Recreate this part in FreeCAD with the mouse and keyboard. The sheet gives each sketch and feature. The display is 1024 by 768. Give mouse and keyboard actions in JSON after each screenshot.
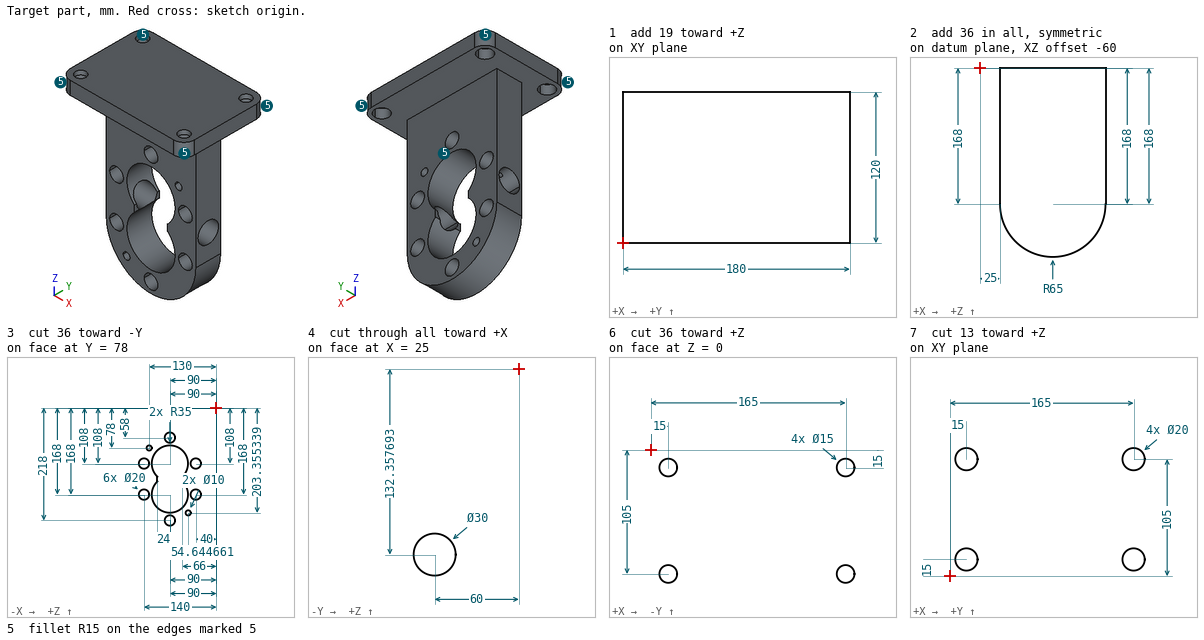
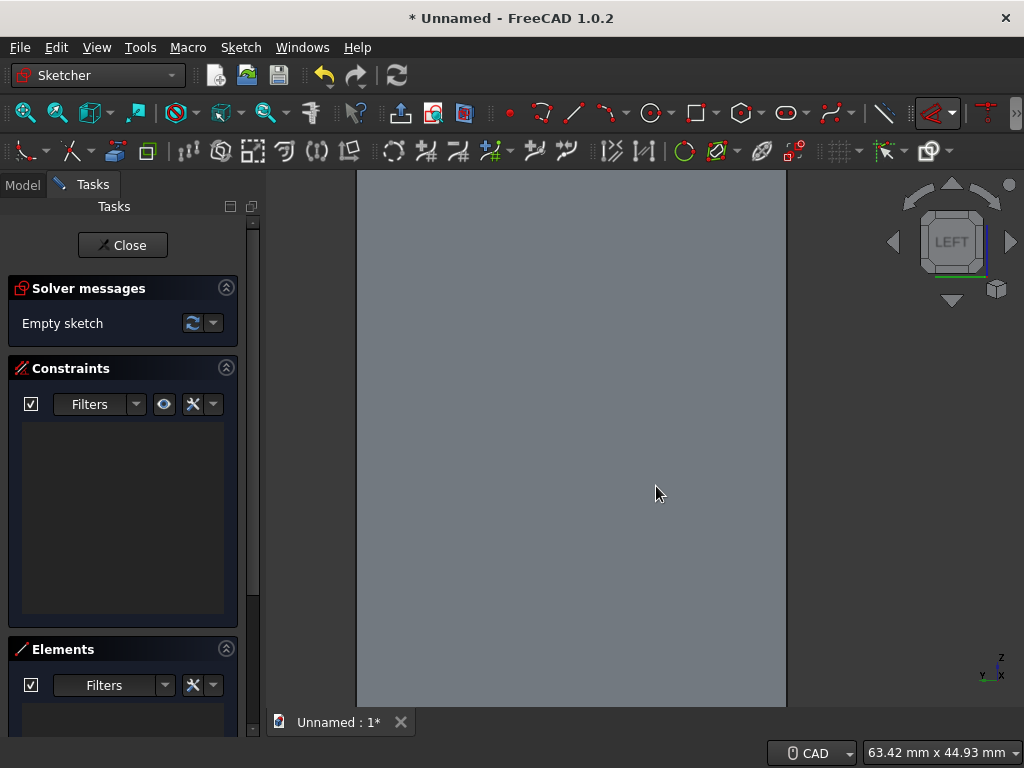
{"action": "left_click", "coordinate": [652, 114]}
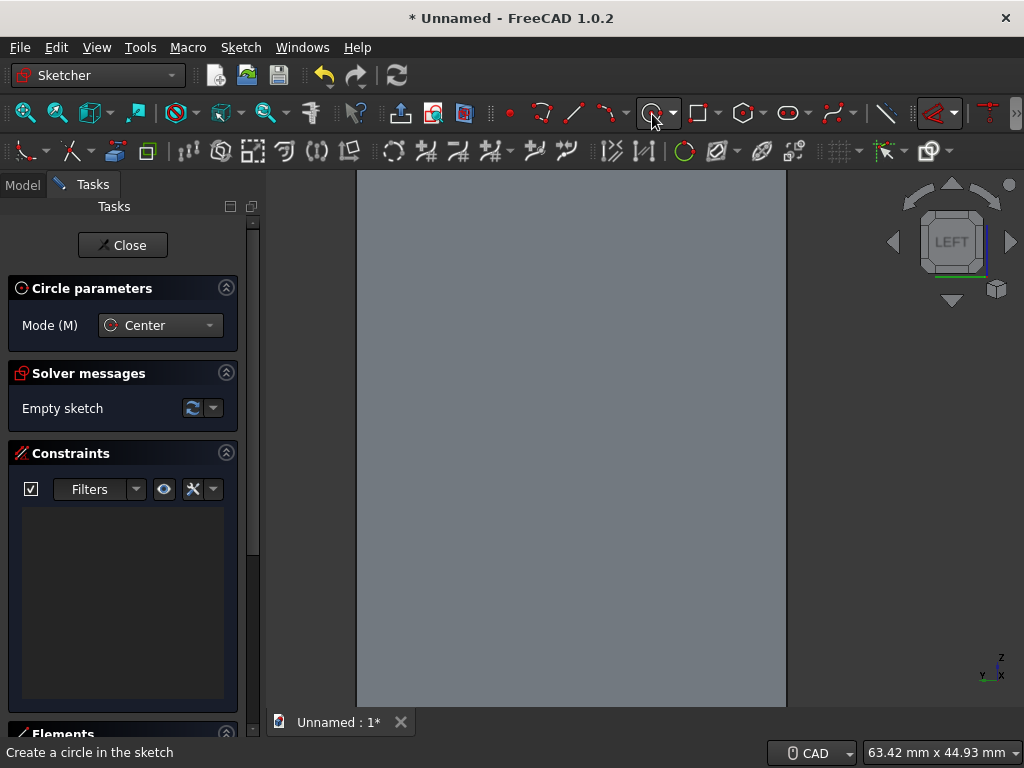
{"action": "left_click", "coordinate": [571, 435]}
{"action": "left_click", "coordinate": [698, 309]}
{"action": "key", "text": "Escape"}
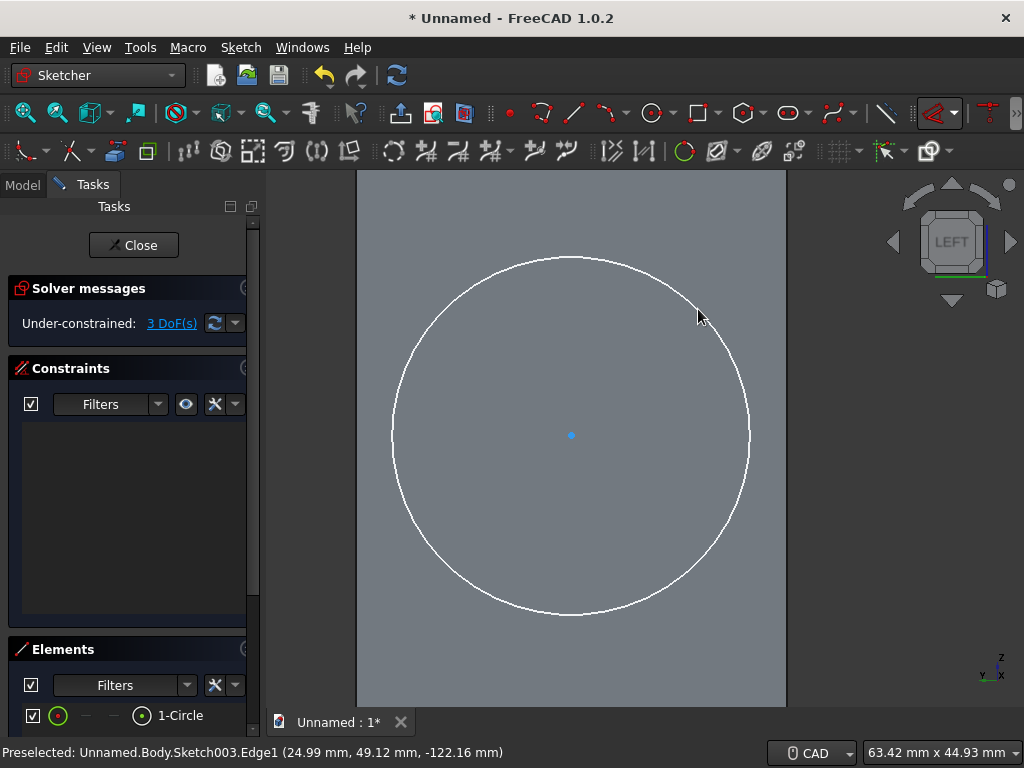
{"action": "left_click", "coordinate": [697, 309]}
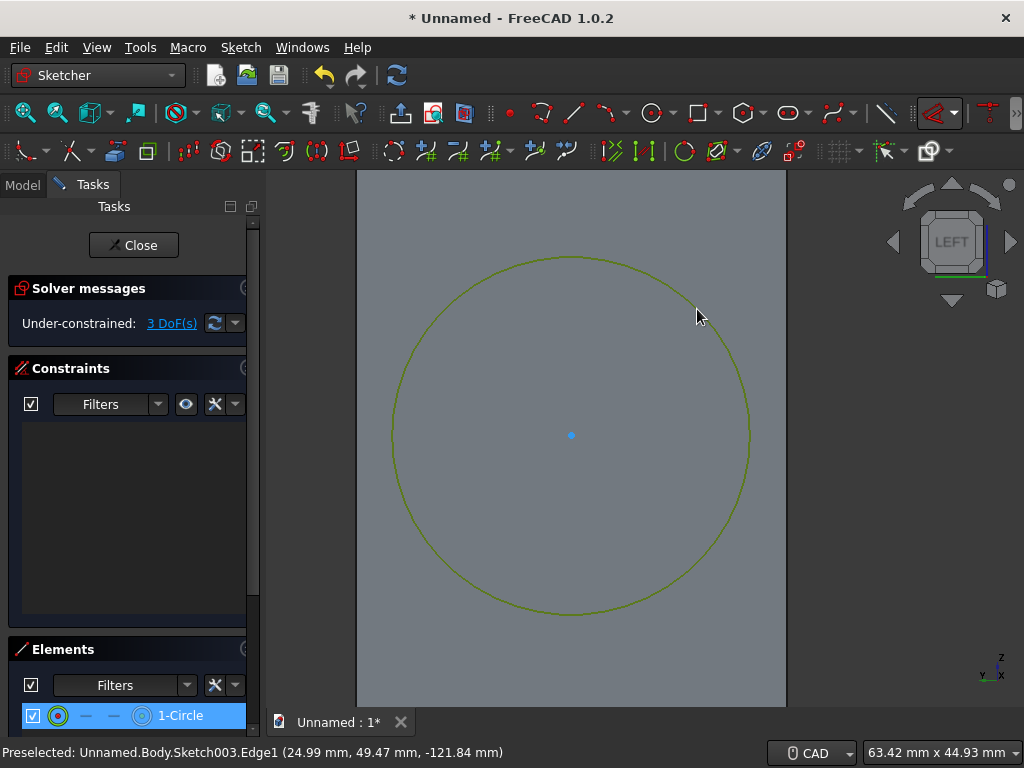
{"action": "left_click", "coordinate": [956, 114]}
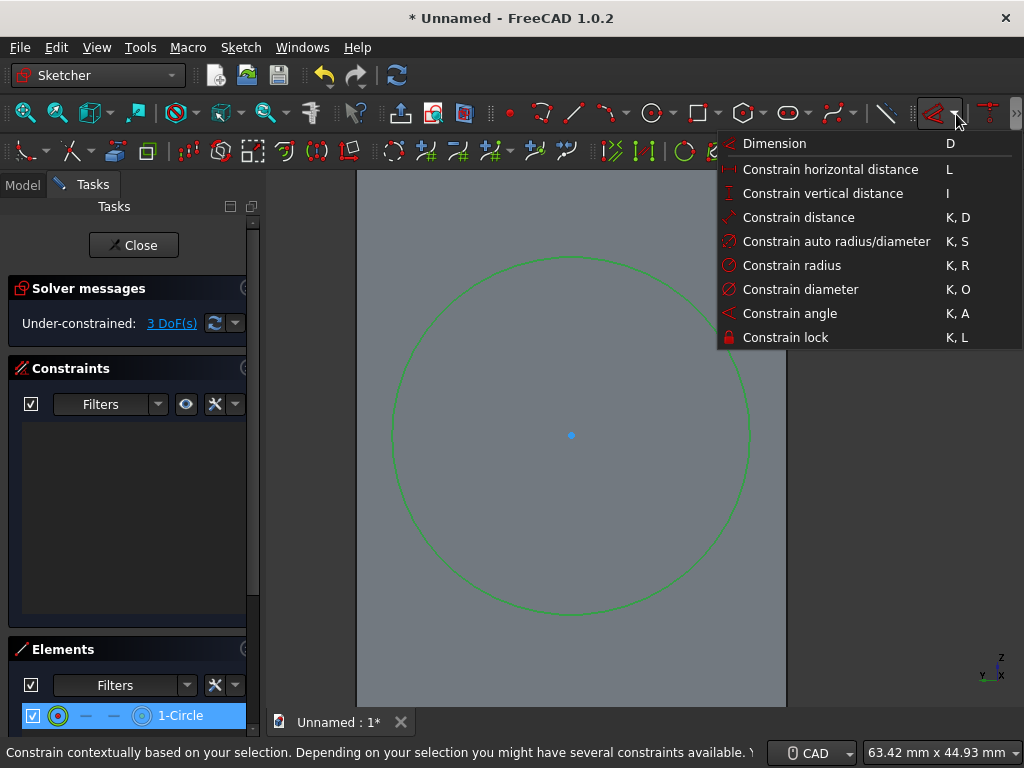
{"action": "left_click", "coordinate": [870, 289]}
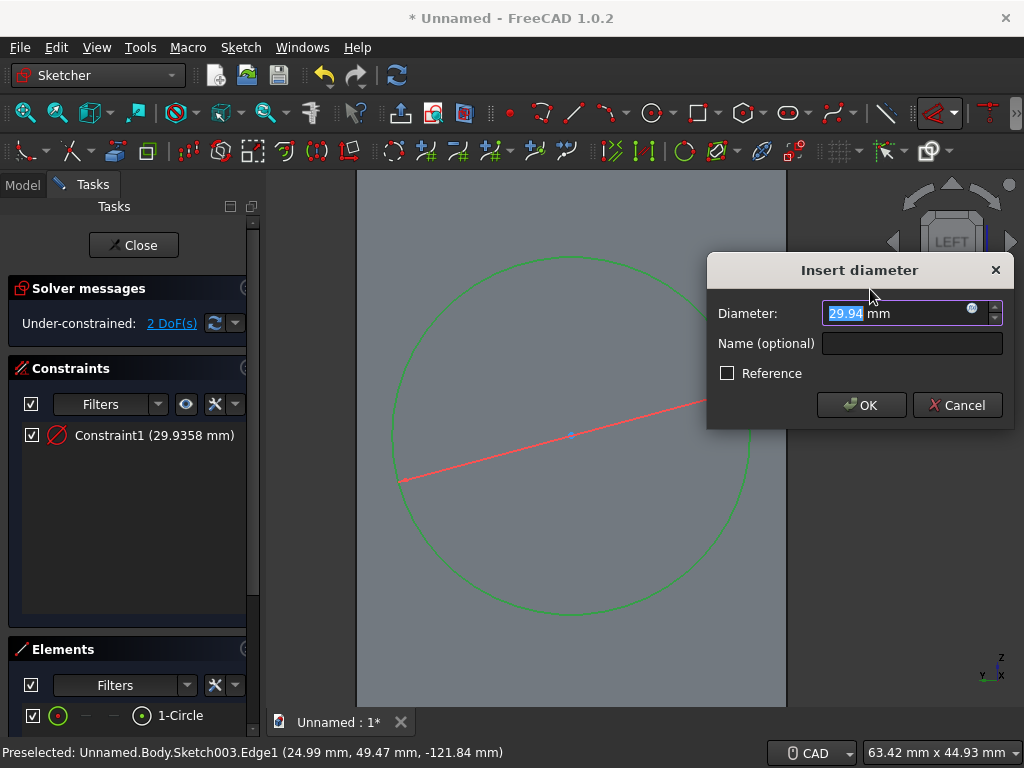
{"action": "type", "text": "30"}
{"action": "key", "text": "Return"}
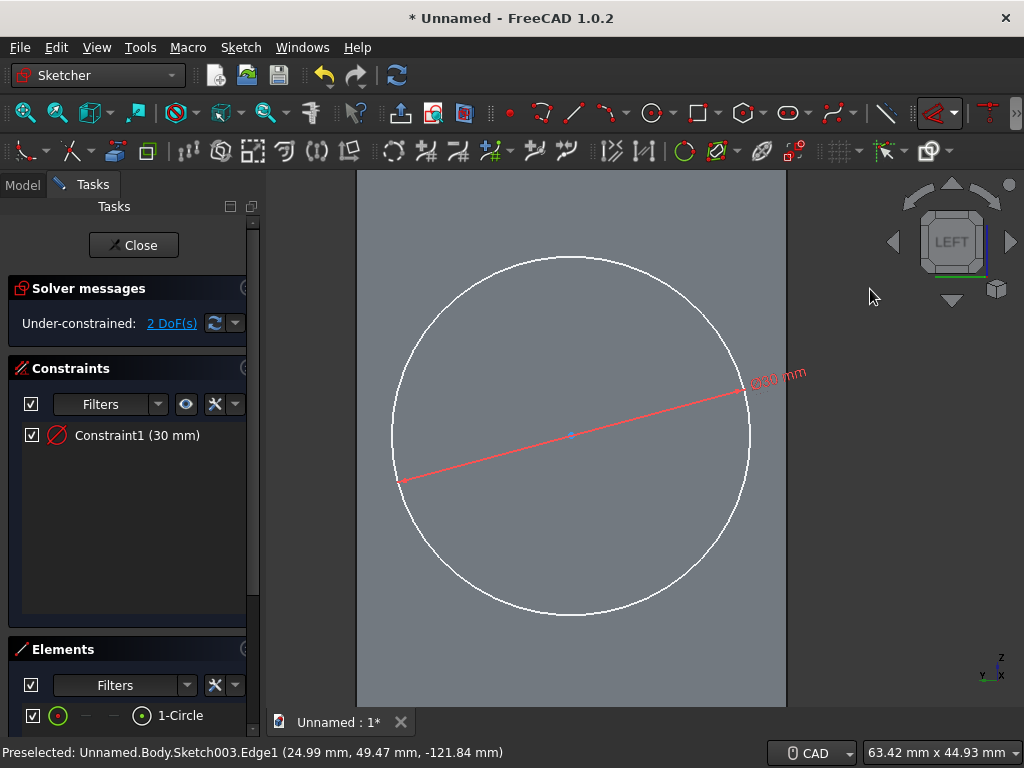
{"action": "left_click", "coordinate": [571, 436]}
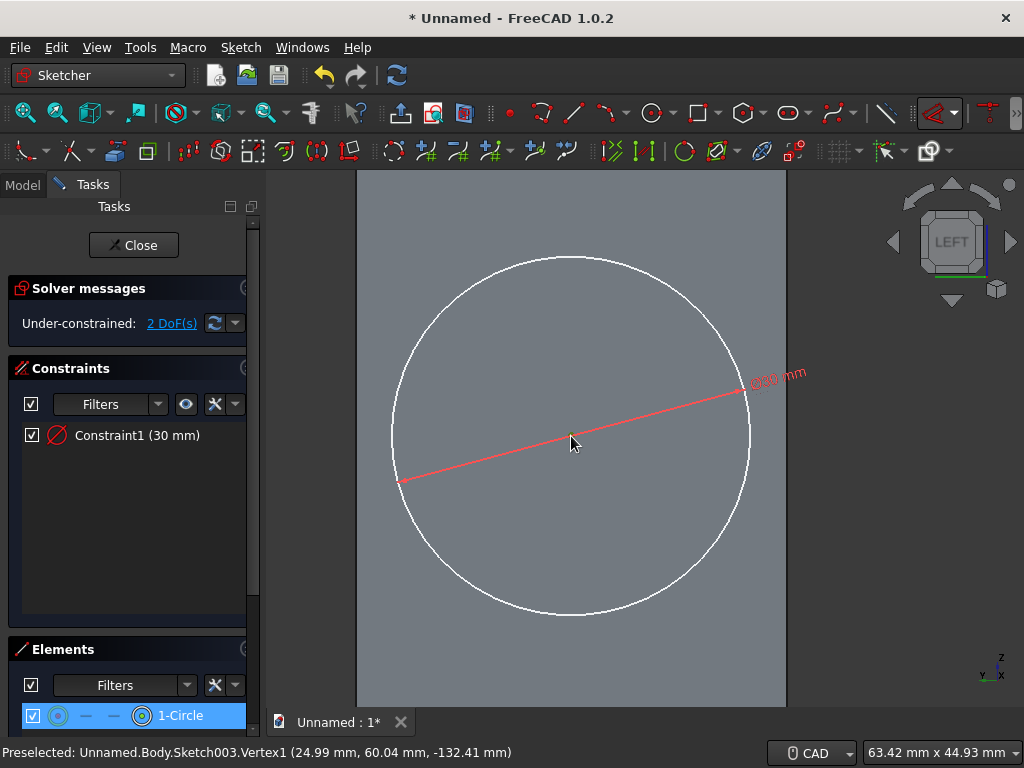
{"action": "key", "text": "l"}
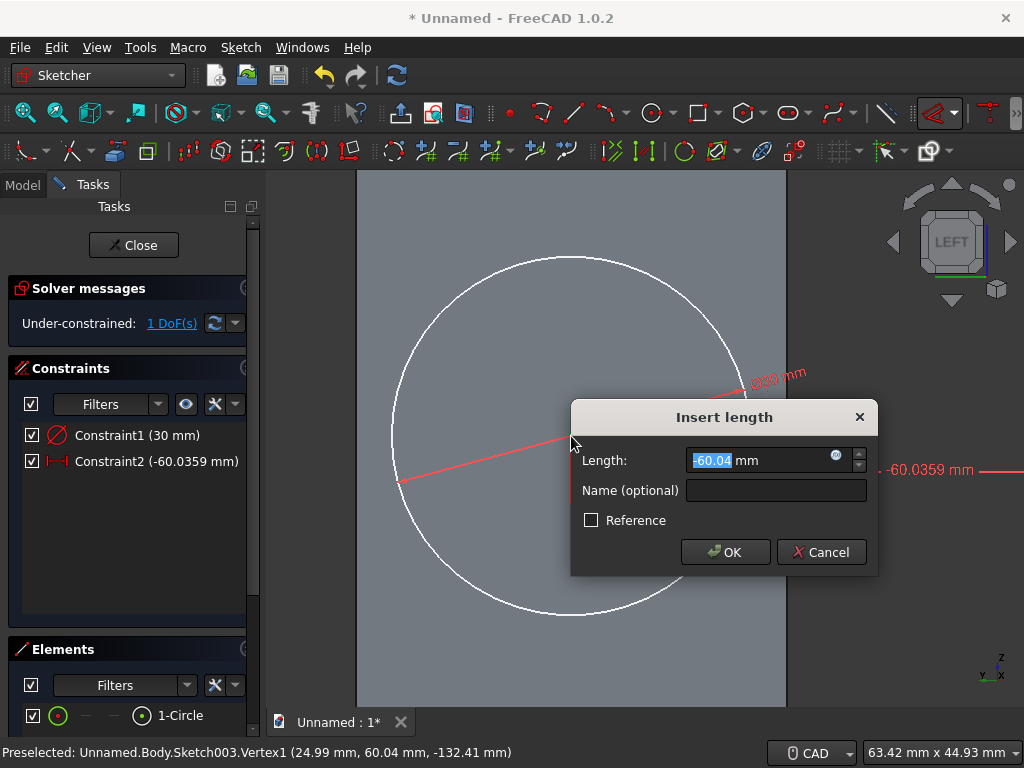
{"action": "type", "text": "-60"}
{"action": "key", "text": "Return"}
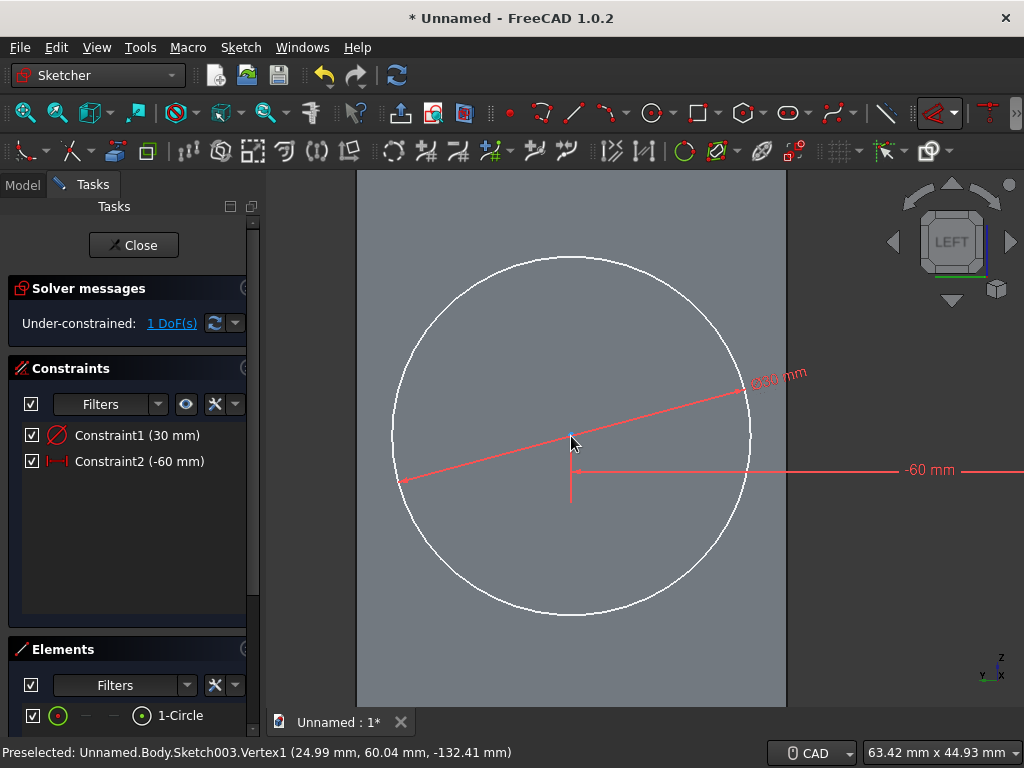
{"action": "left_click", "coordinate": [571, 436]}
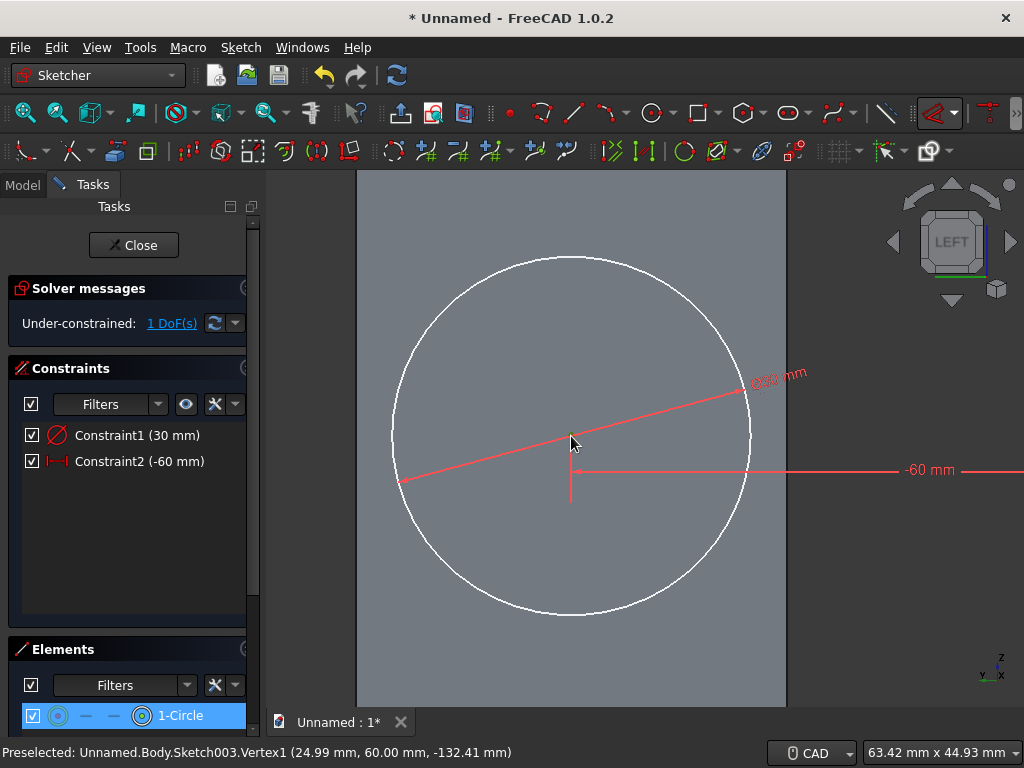
{"action": "left_click", "coordinate": [956, 114]}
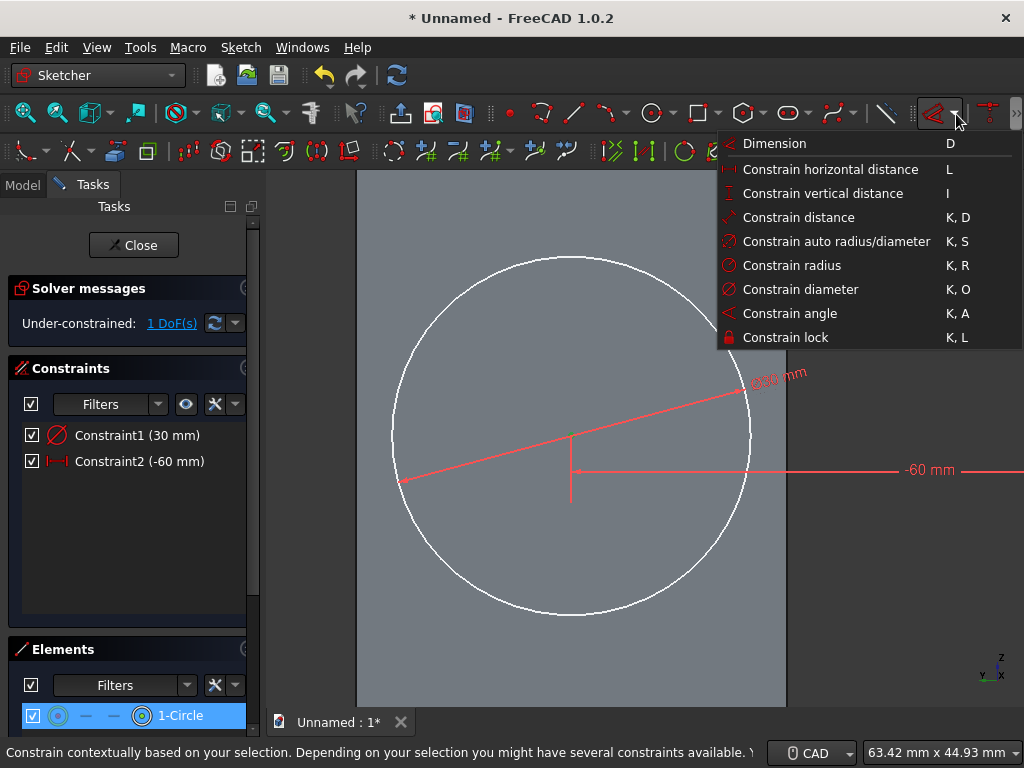
{"action": "left_click", "coordinate": [870, 193]}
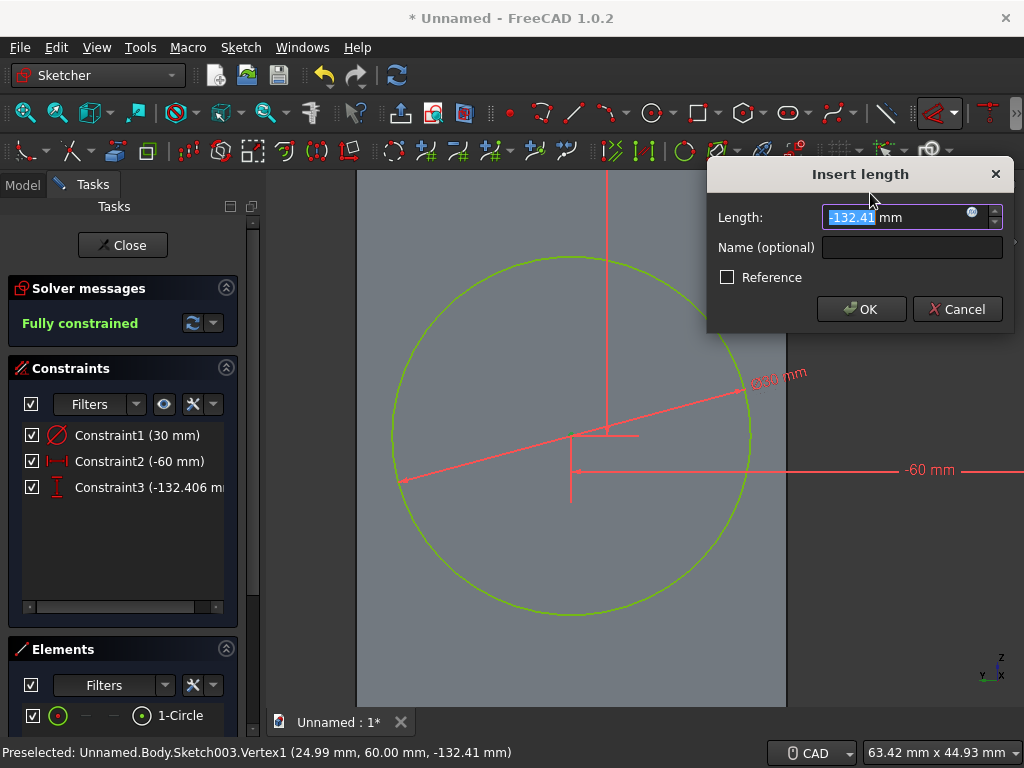
{"action": "type", "text": "-132.357693"}
{"action": "key", "text": "Return"}